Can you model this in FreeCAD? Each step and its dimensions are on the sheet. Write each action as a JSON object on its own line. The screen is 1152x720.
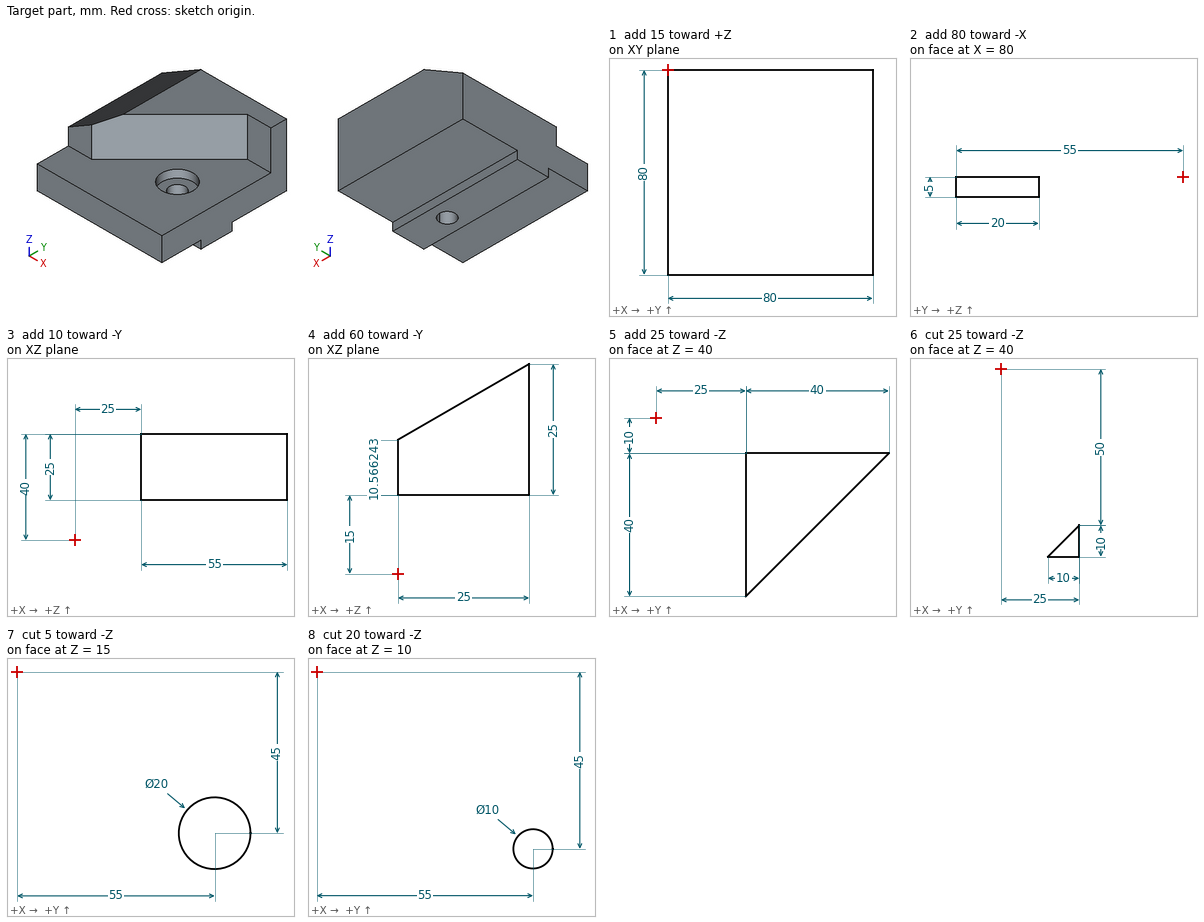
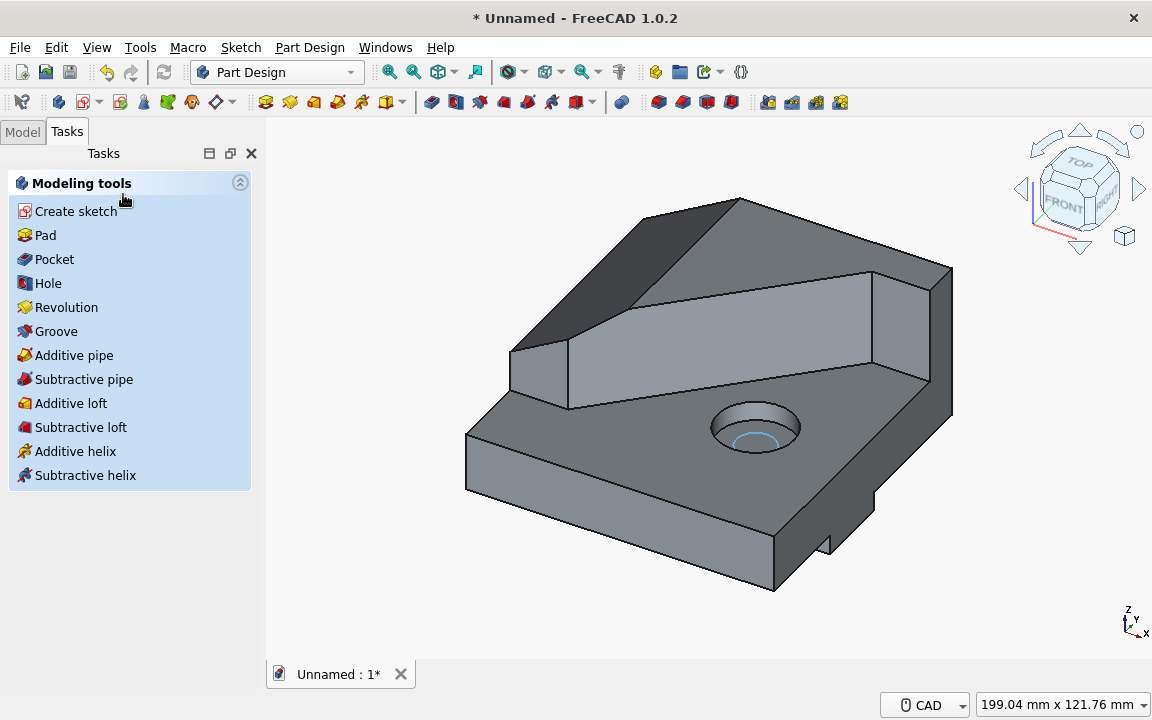
{"action": "left_click", "coordinate": [432, 102]}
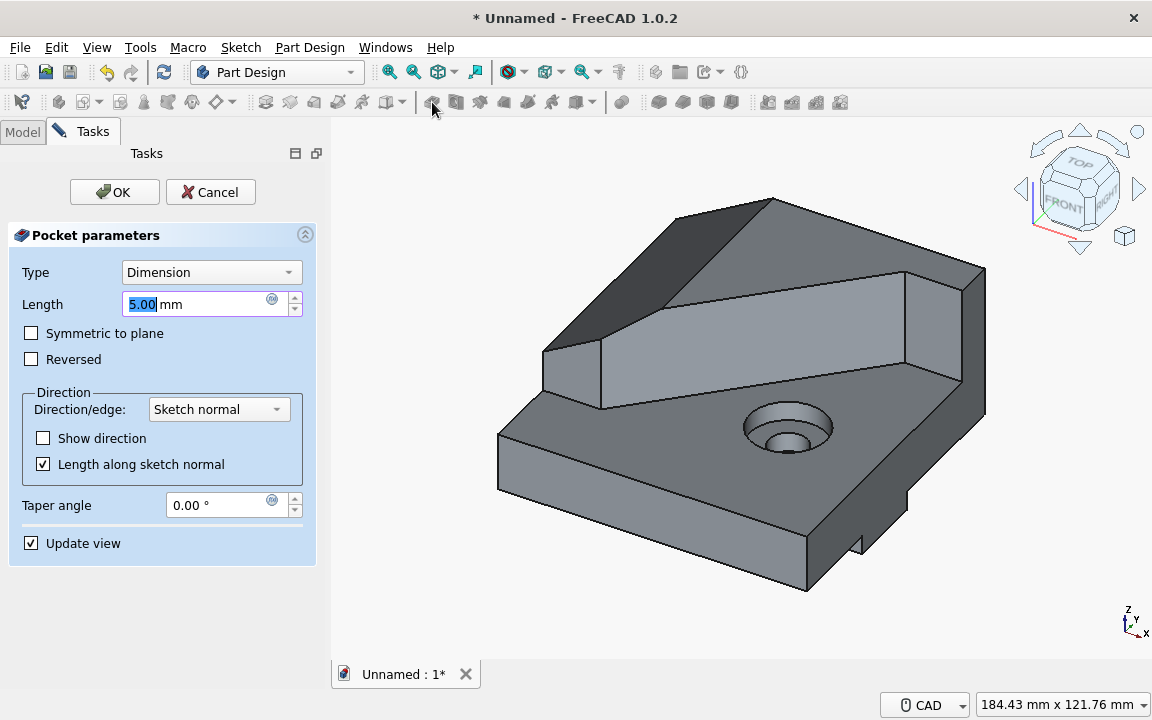
{"action": "type", "text": "20"}
{"action": "key", "text": "Tab"}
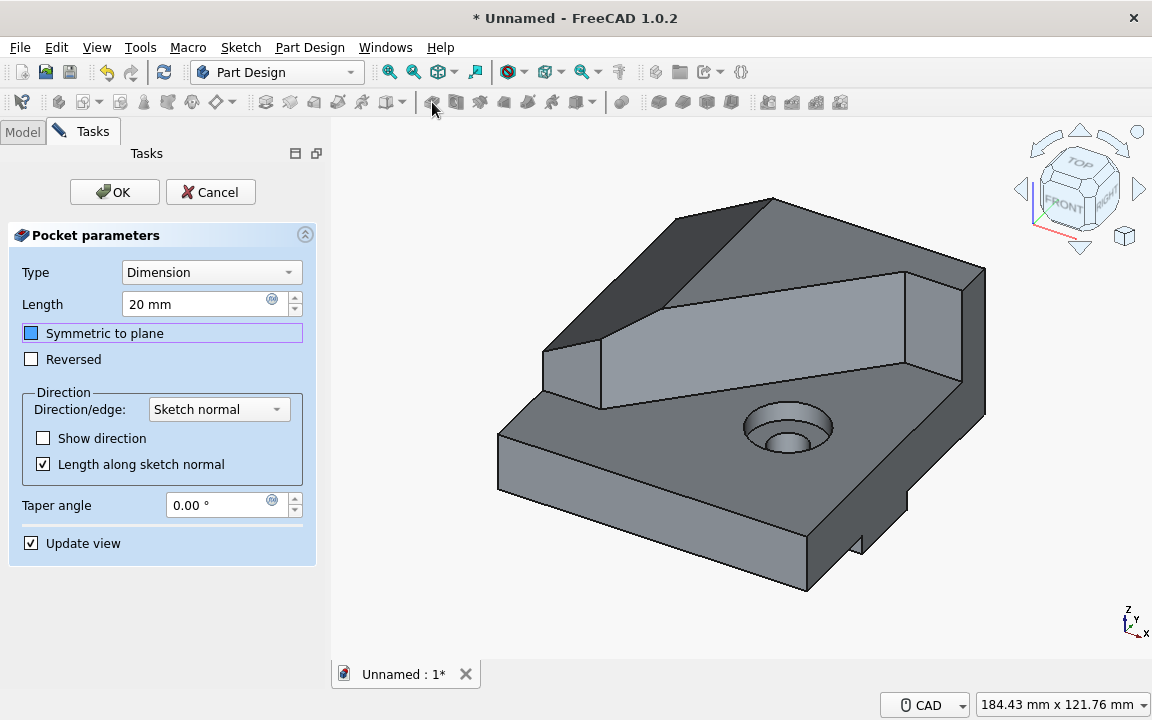
{"action": "left_click", "coordinate": [115, 192]}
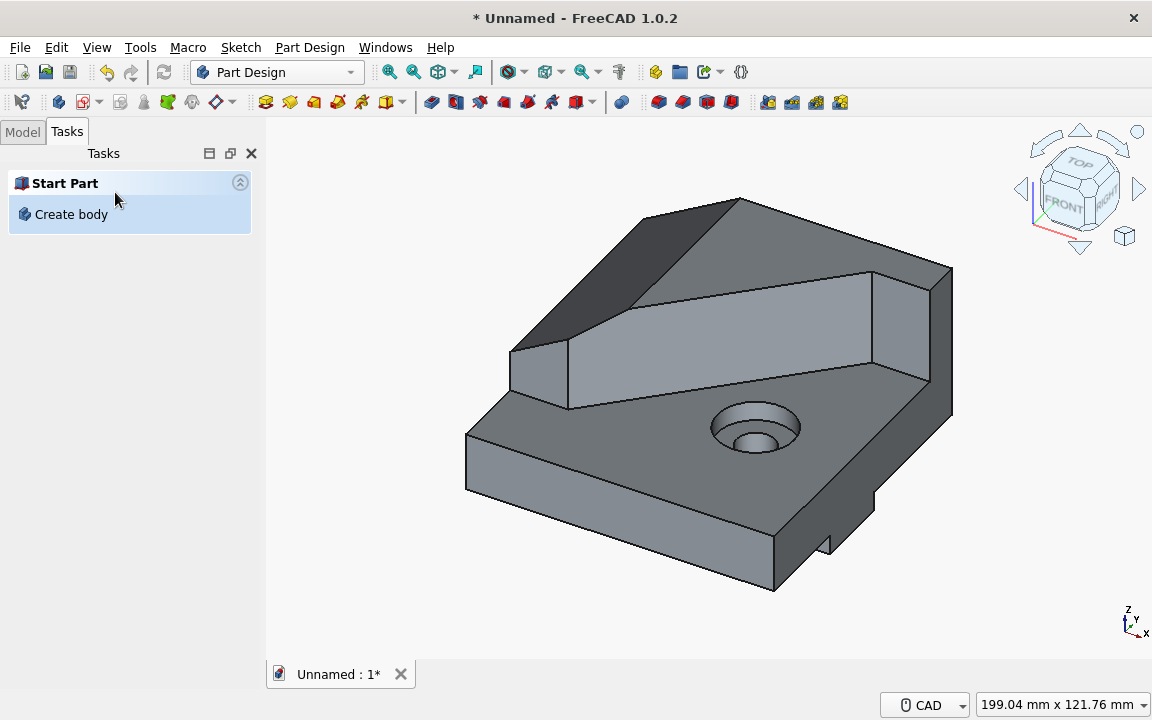
{"action": "key", "text": "0"}